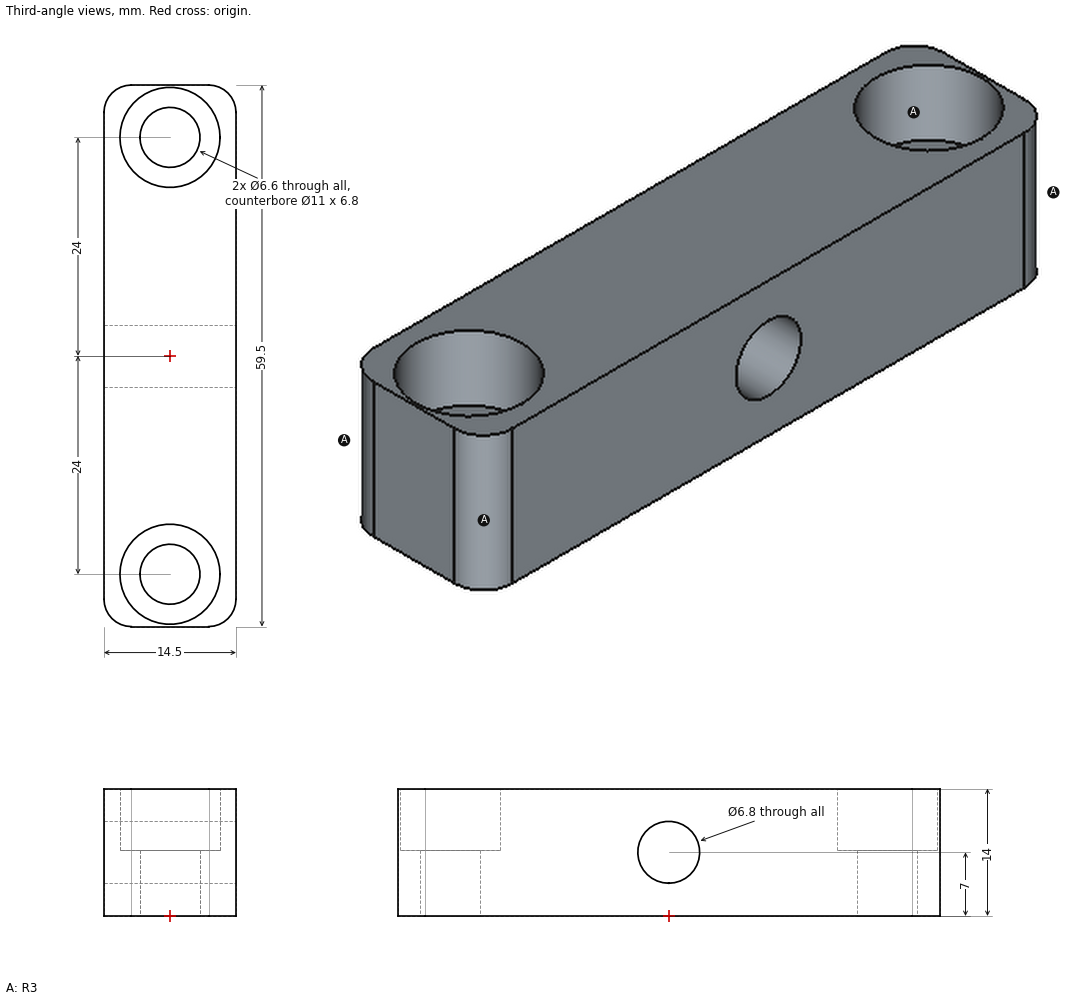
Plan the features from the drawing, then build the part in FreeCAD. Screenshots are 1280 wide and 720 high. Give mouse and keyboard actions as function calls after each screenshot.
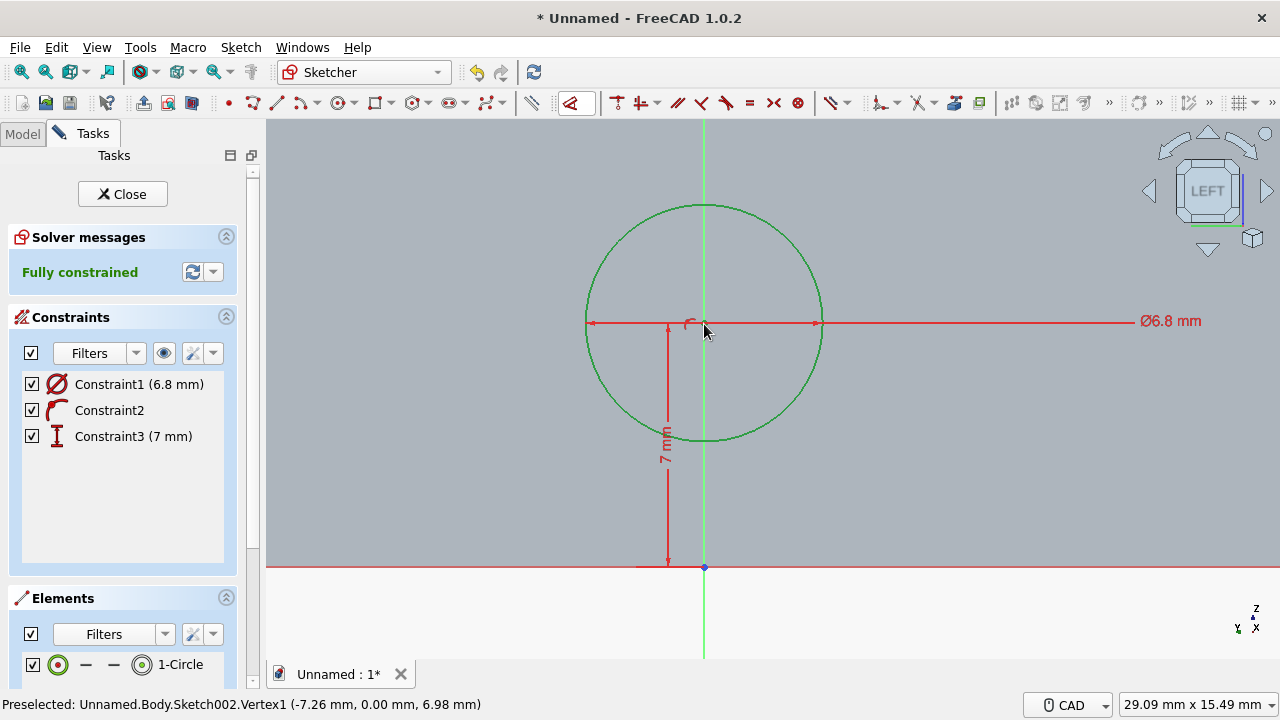
click(123, 194)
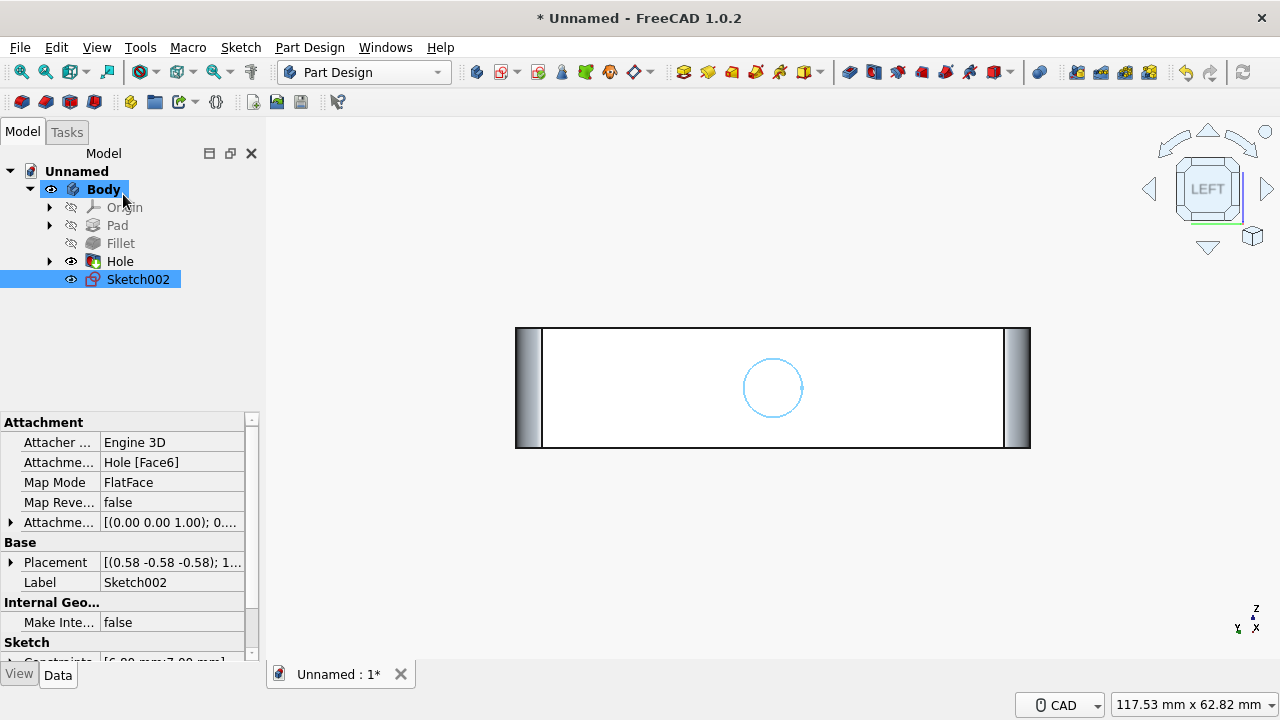
click(874, 72)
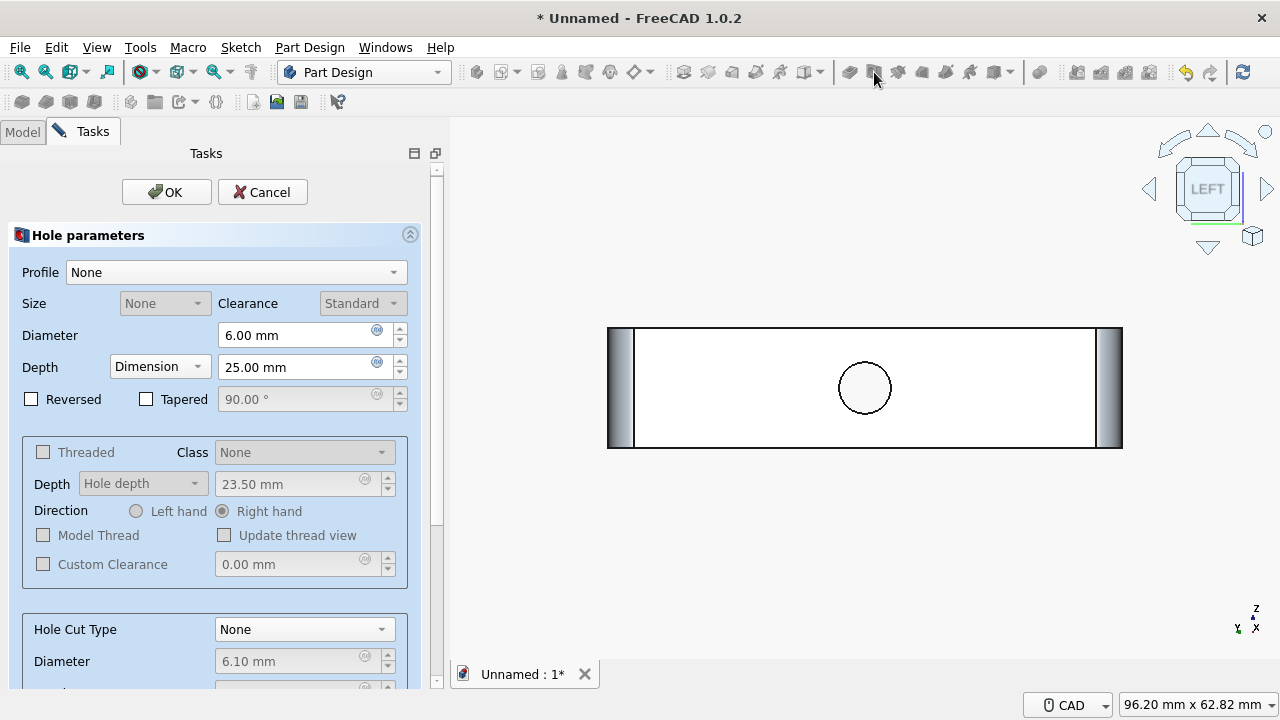
triple_click(305, 335)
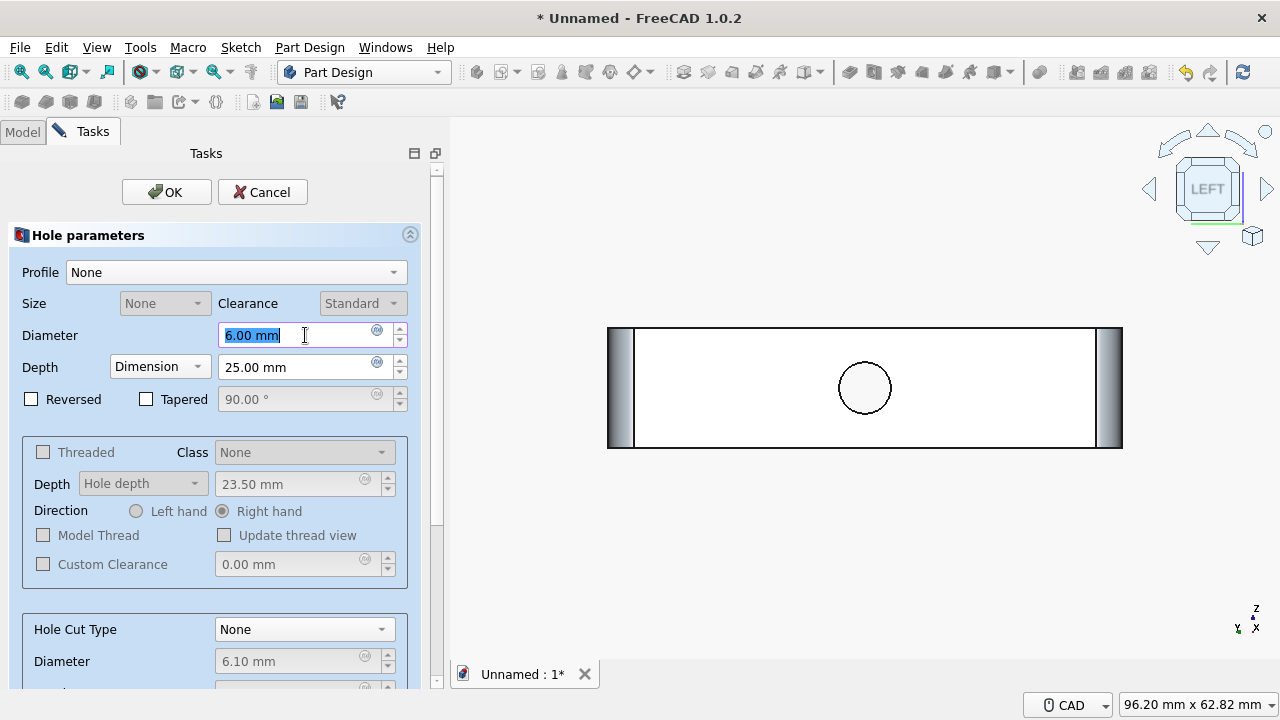
text(6.8)
key(Tab)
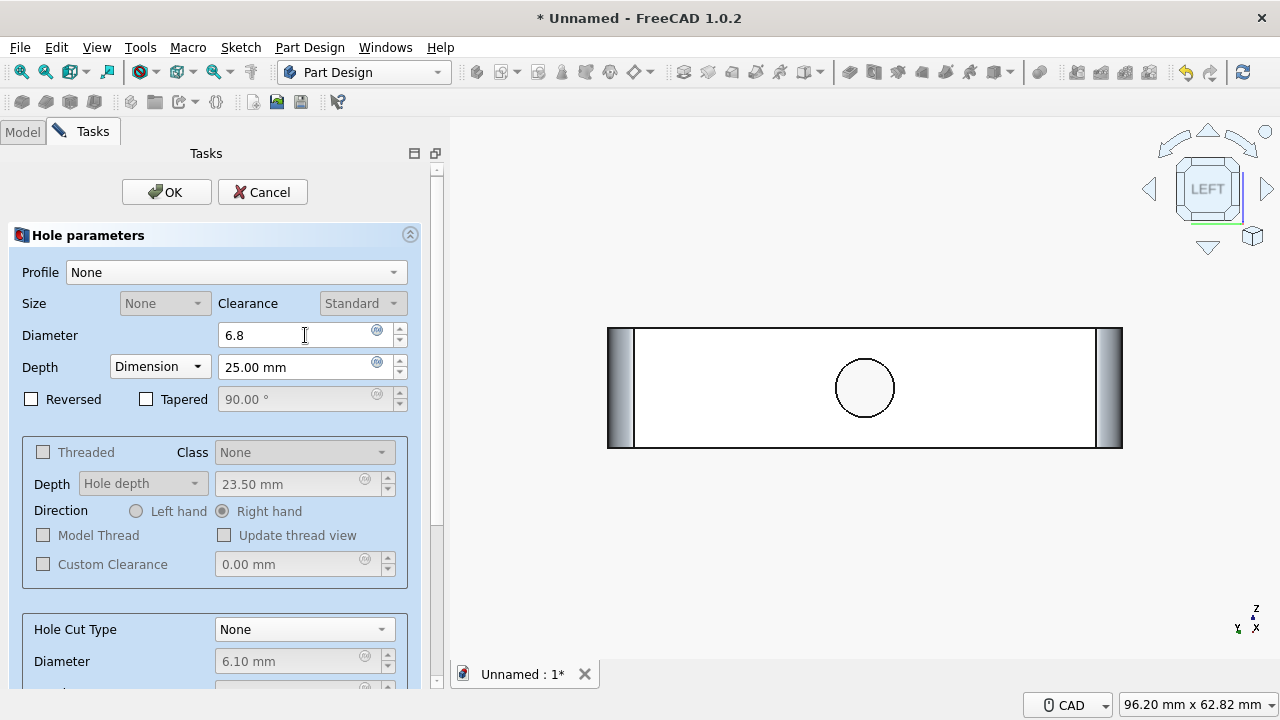
click(161, 366)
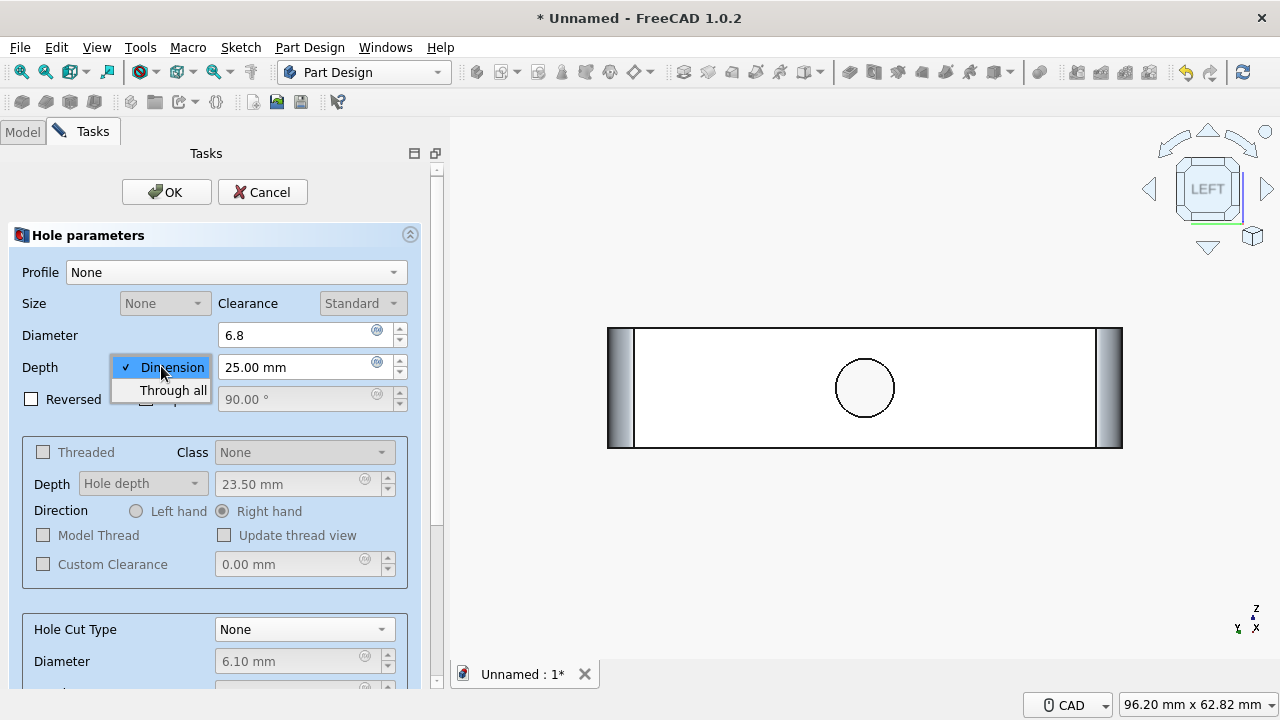
click(160, 390)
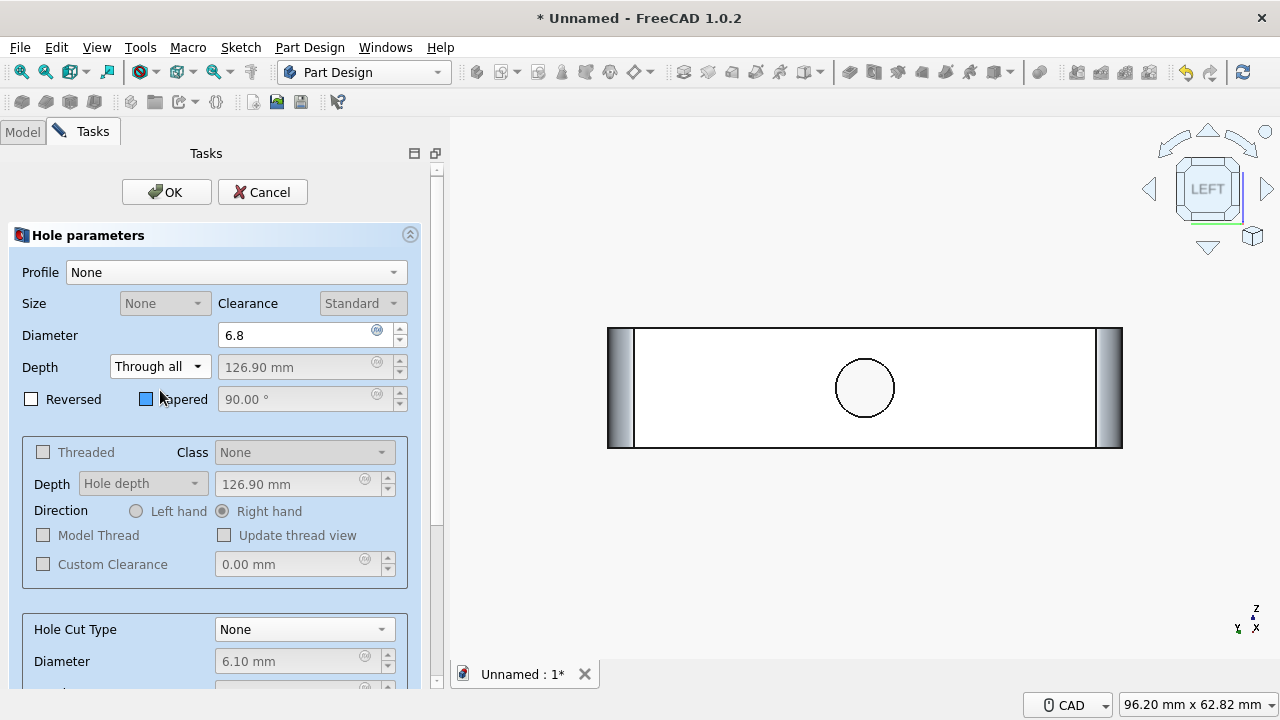
click(167, 192)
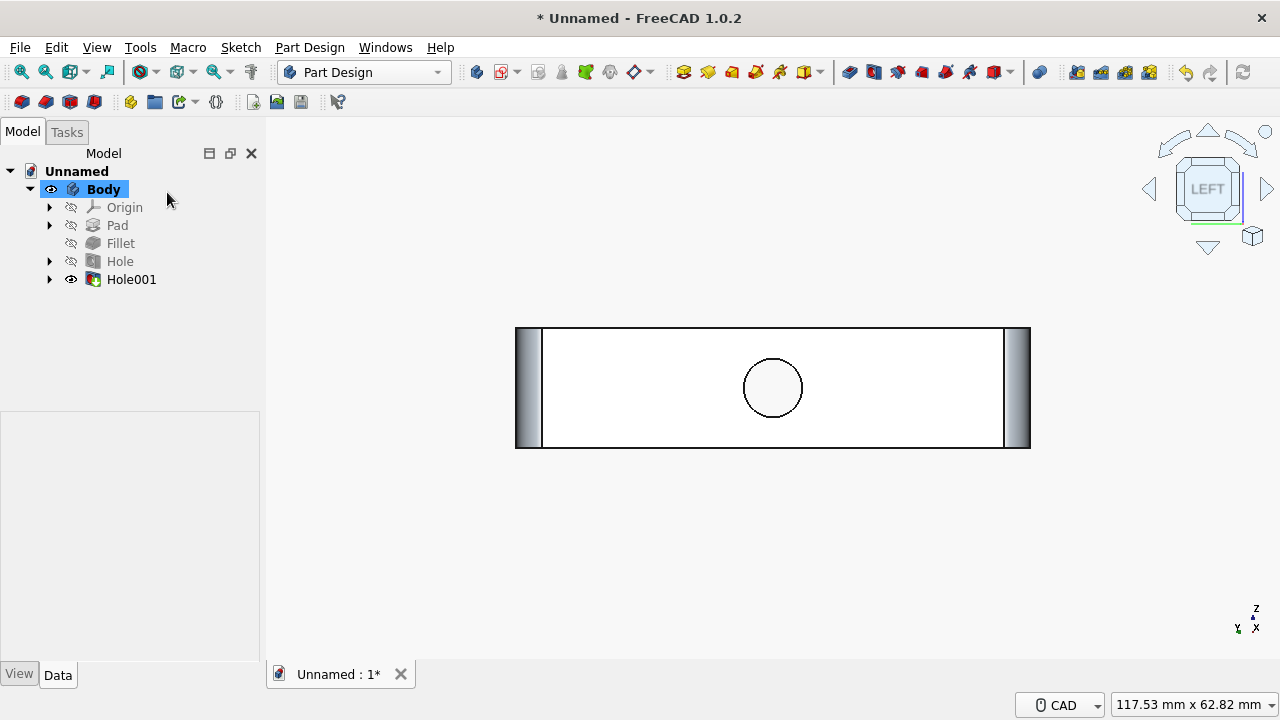
key(0)